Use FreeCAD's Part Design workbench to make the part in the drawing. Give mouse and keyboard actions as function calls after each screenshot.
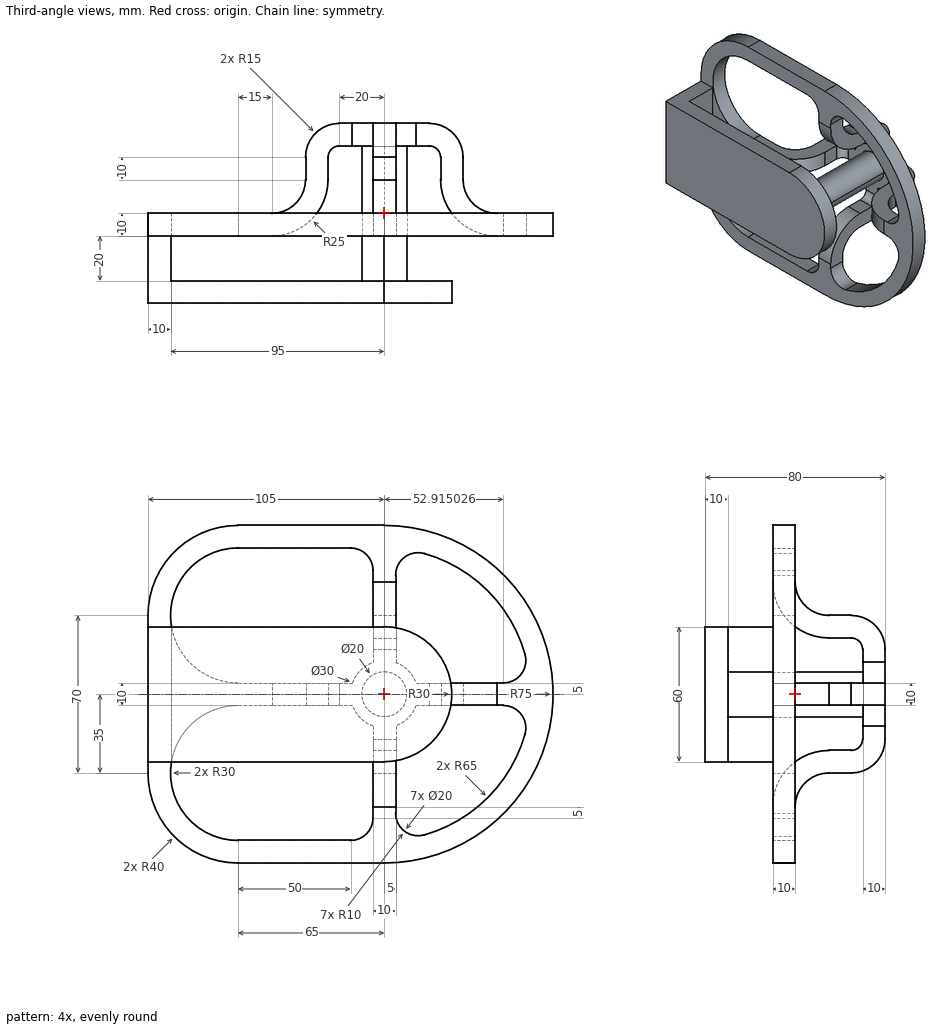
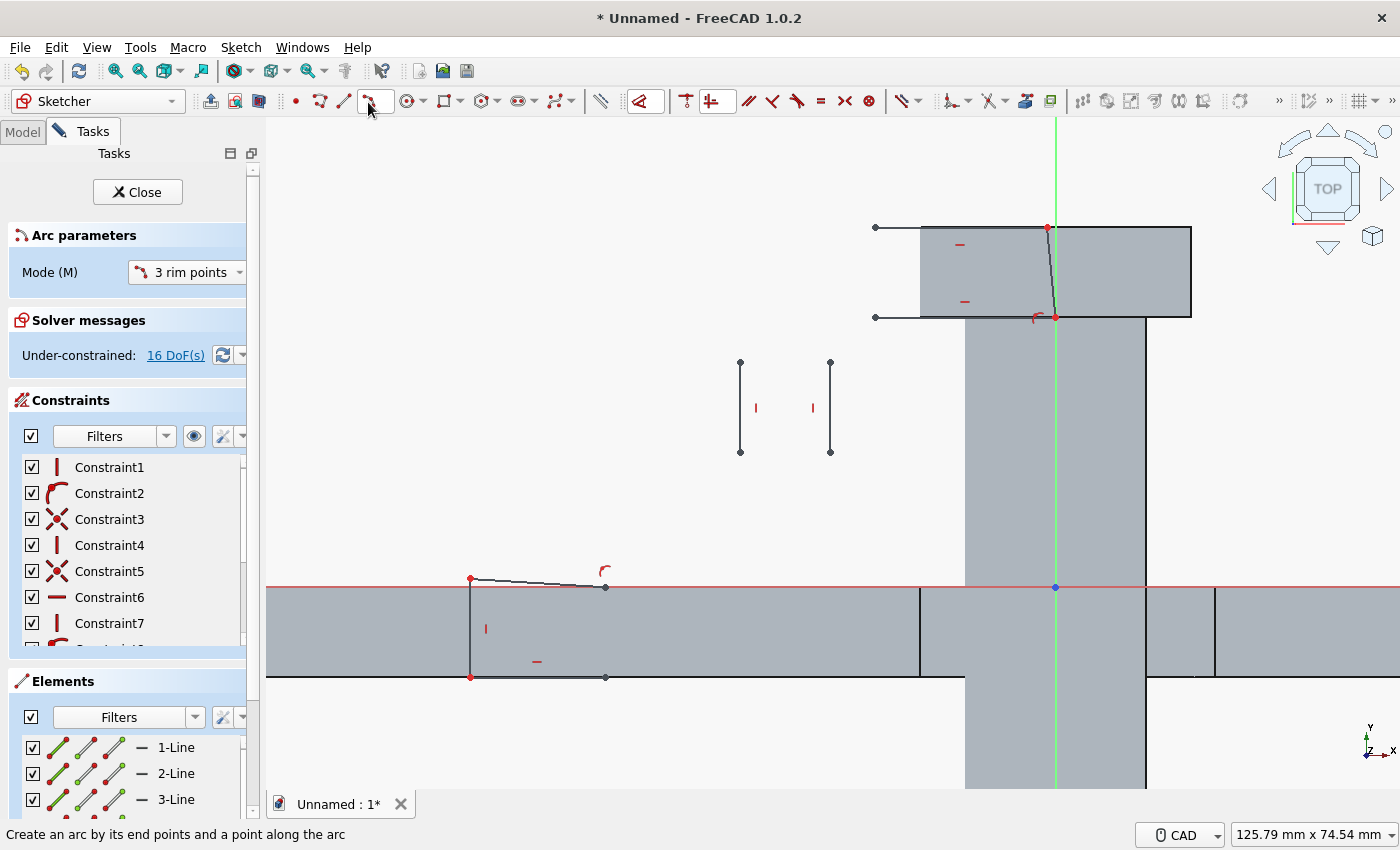
click(740, 453)
click(605, 587)
click(700, 548)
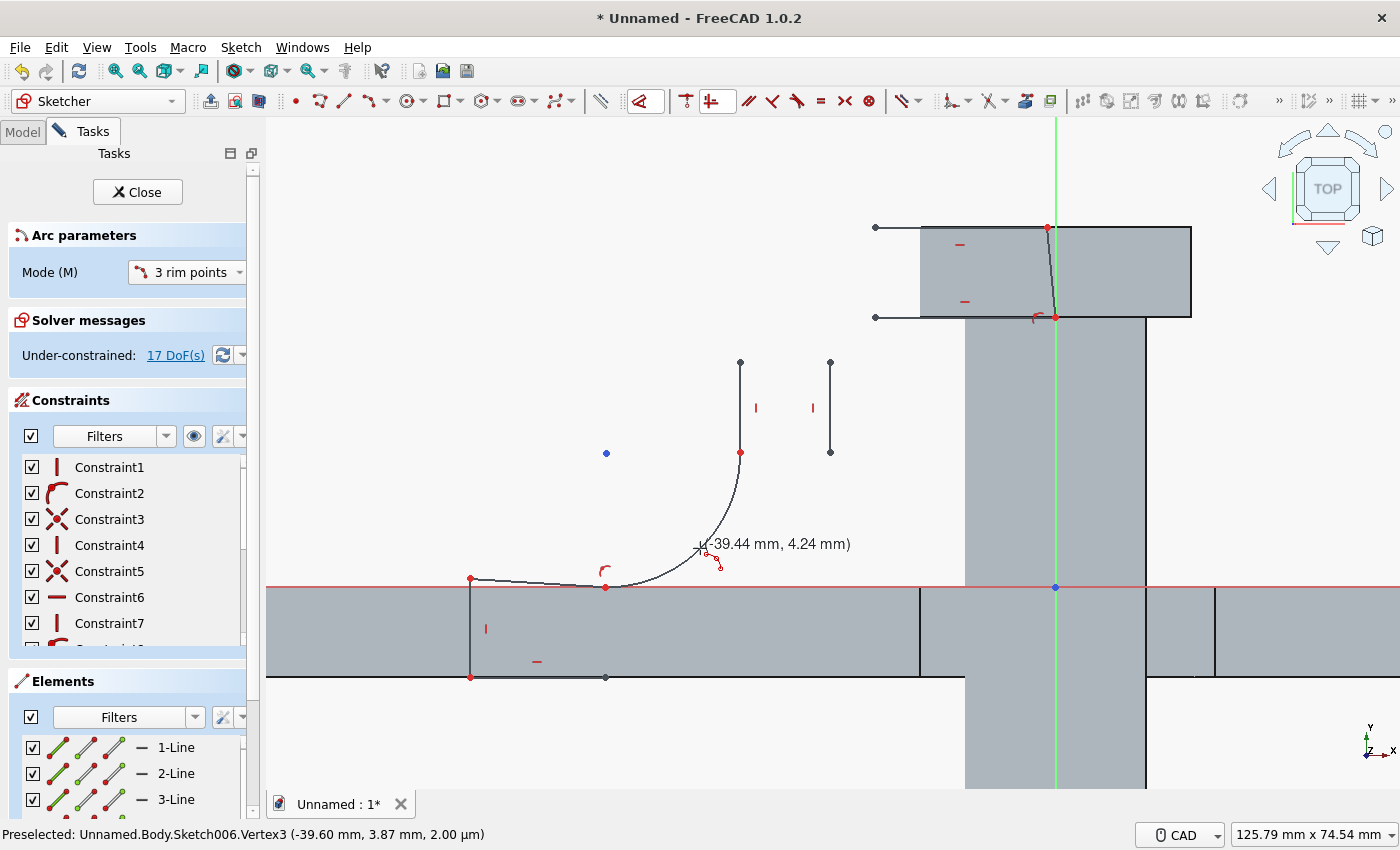
click(605, 678)
click(830, 453)
click(764, 611)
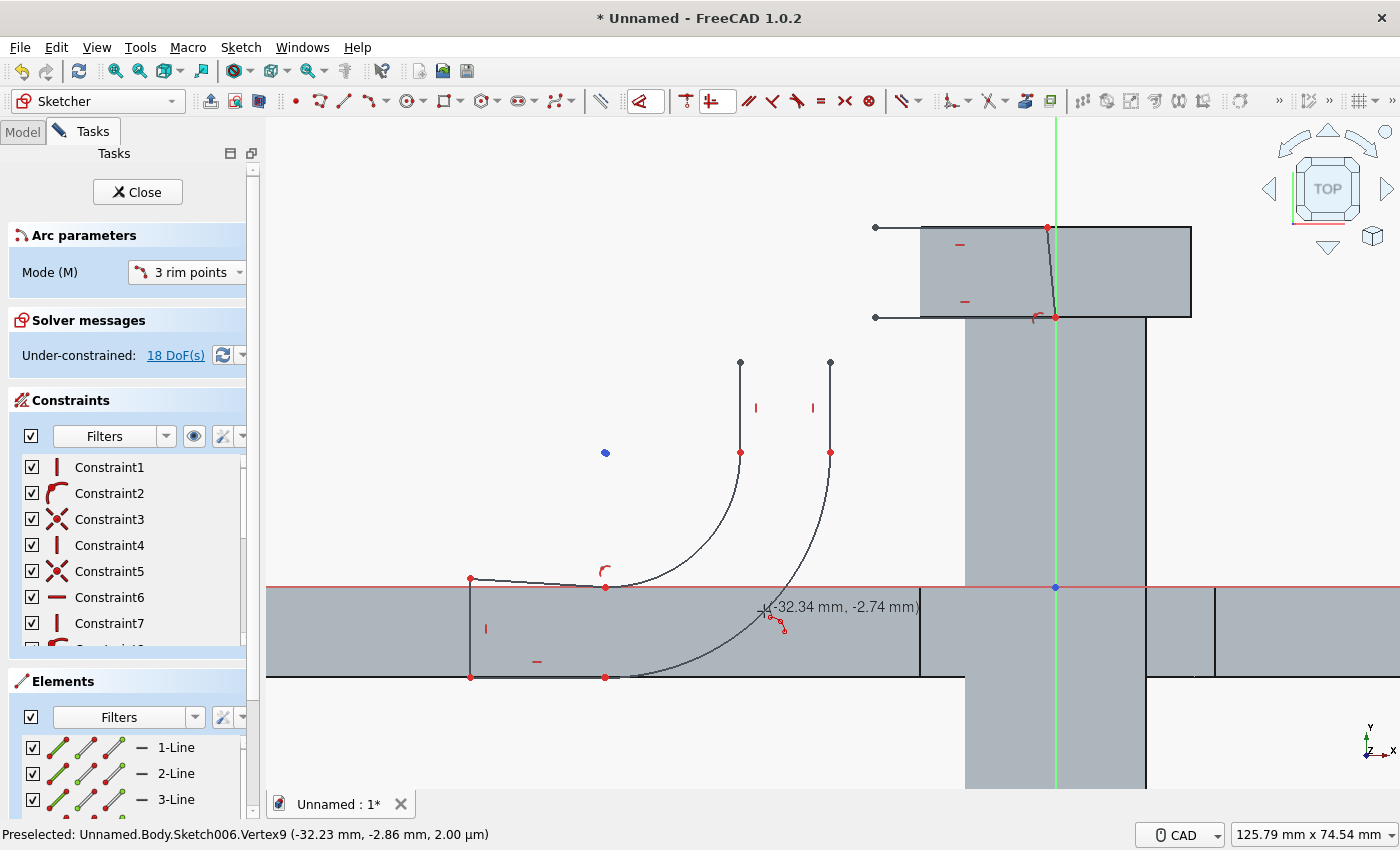
click(830, 363)
click(875, 318)
click(843, 330)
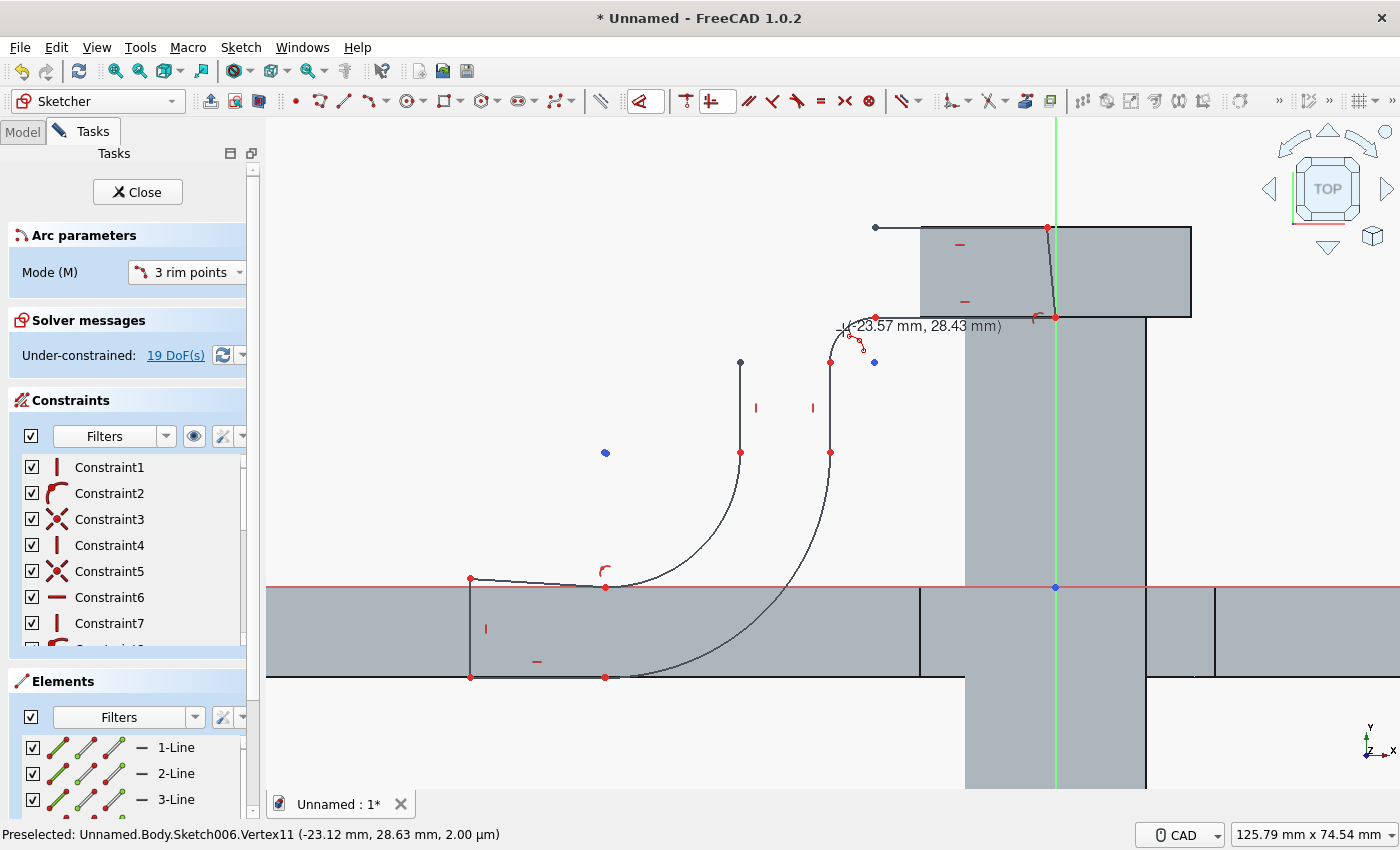
click(875, 228)
click(740, 363)
click(780, 266)
key(Escape)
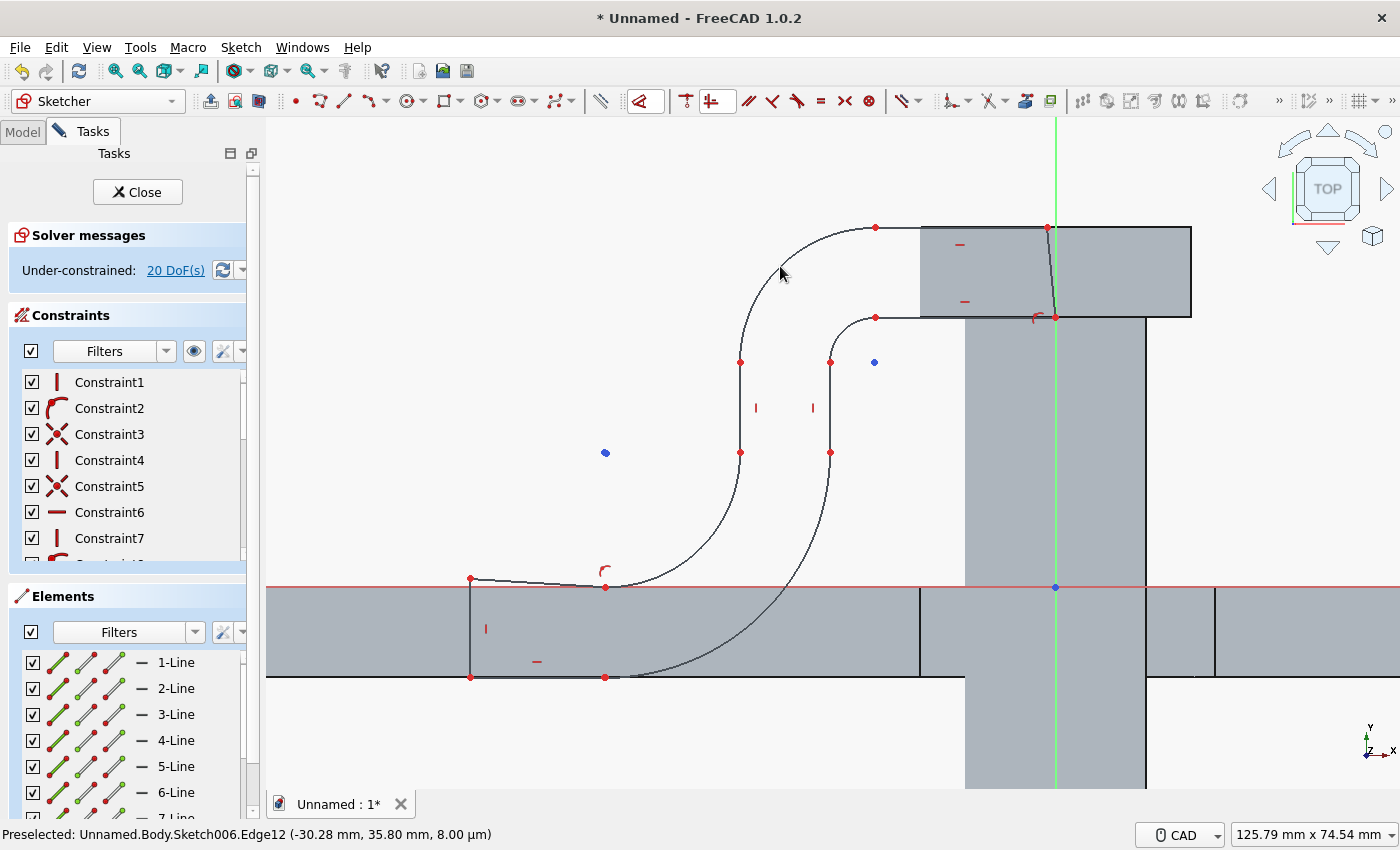
click(740, 390)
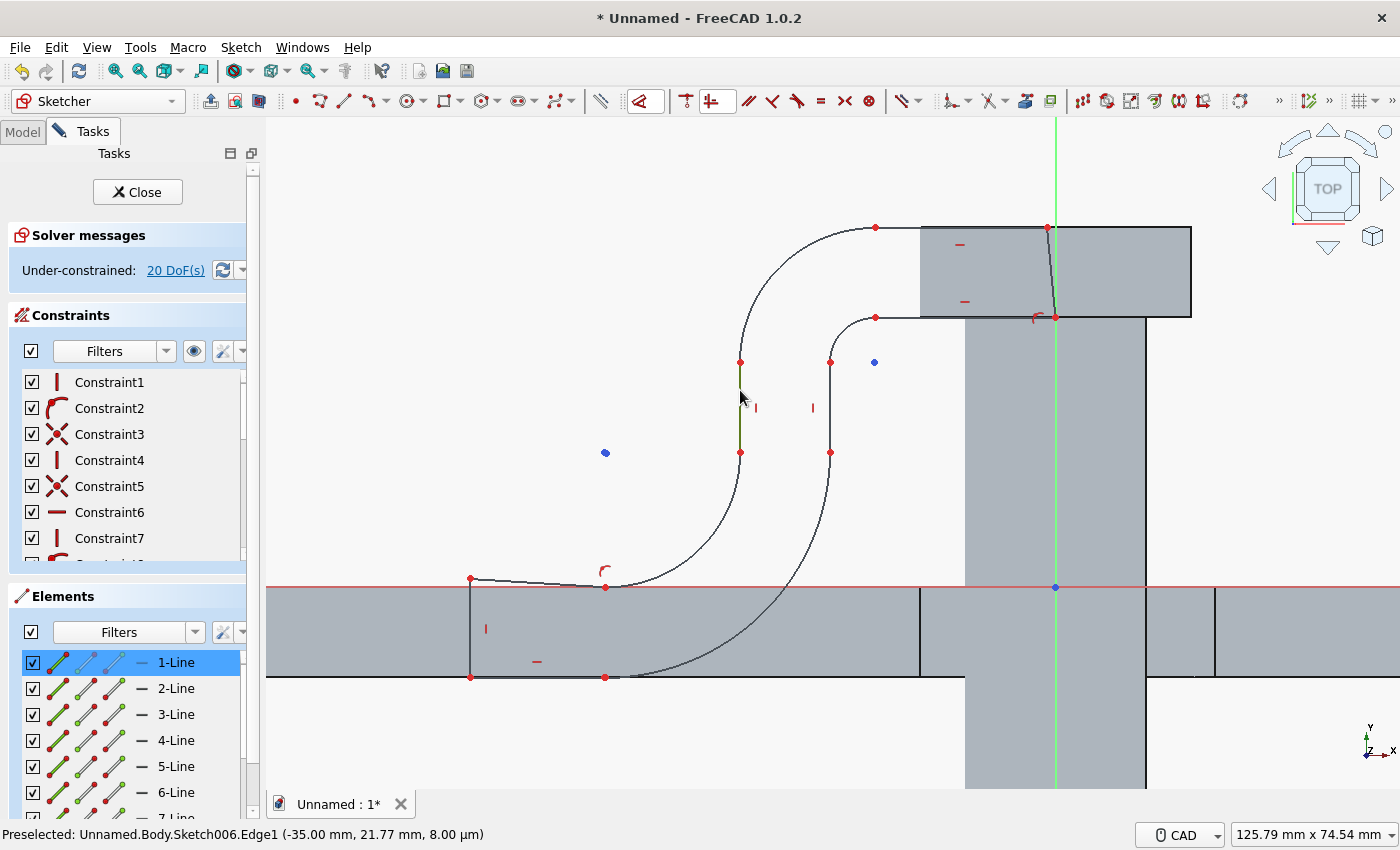
click(666, 573)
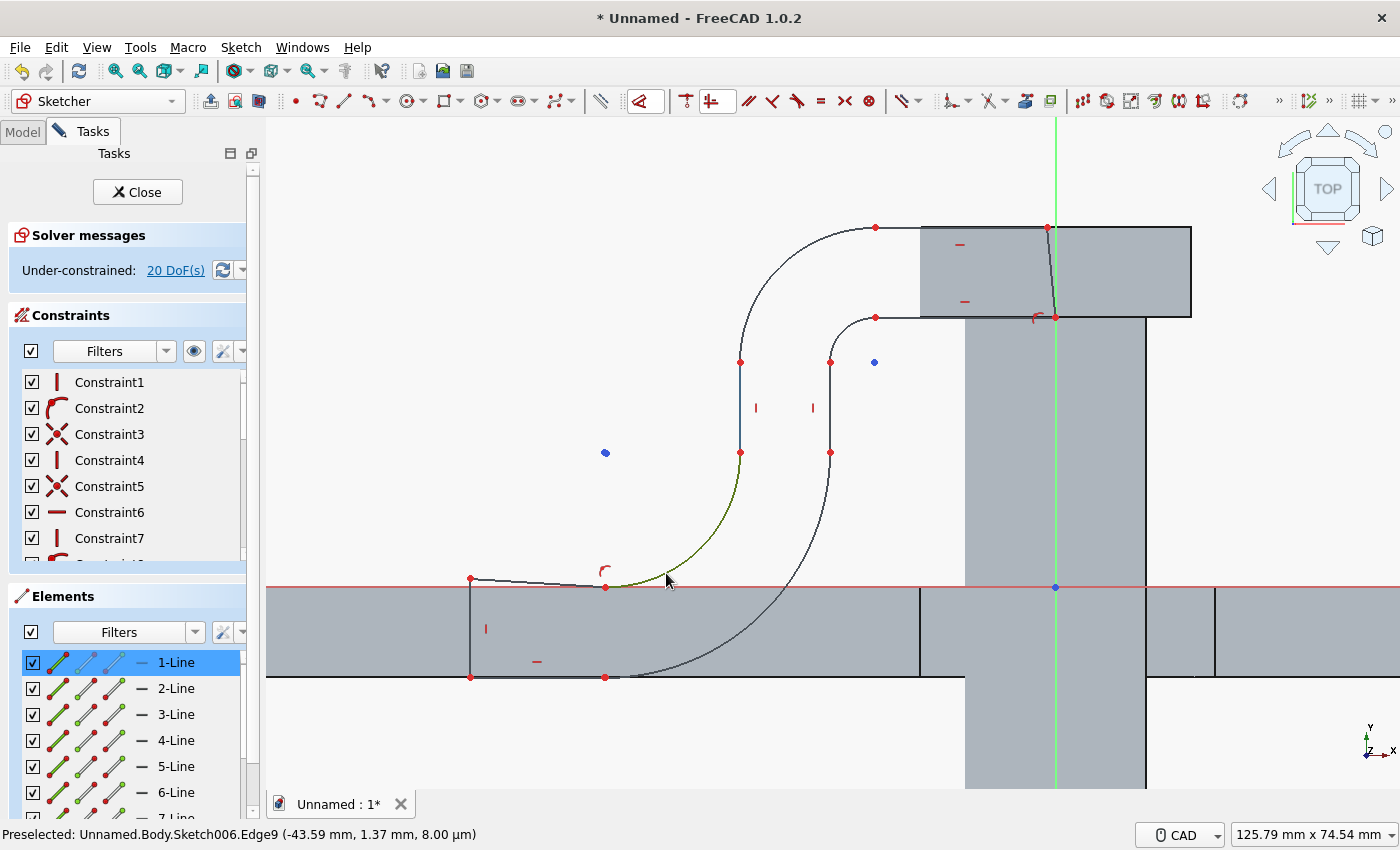
click(798, 102)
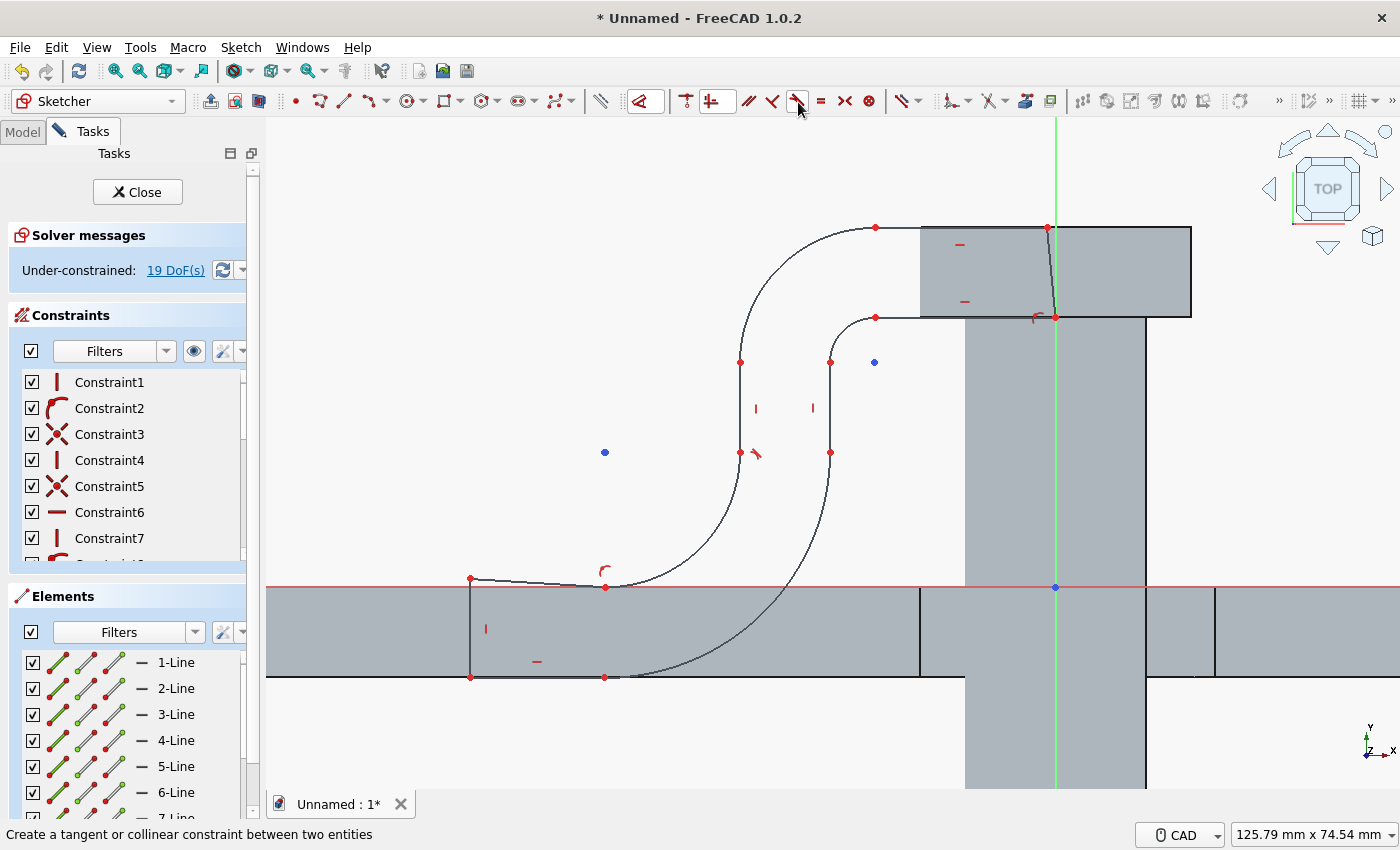
click(740, 390)